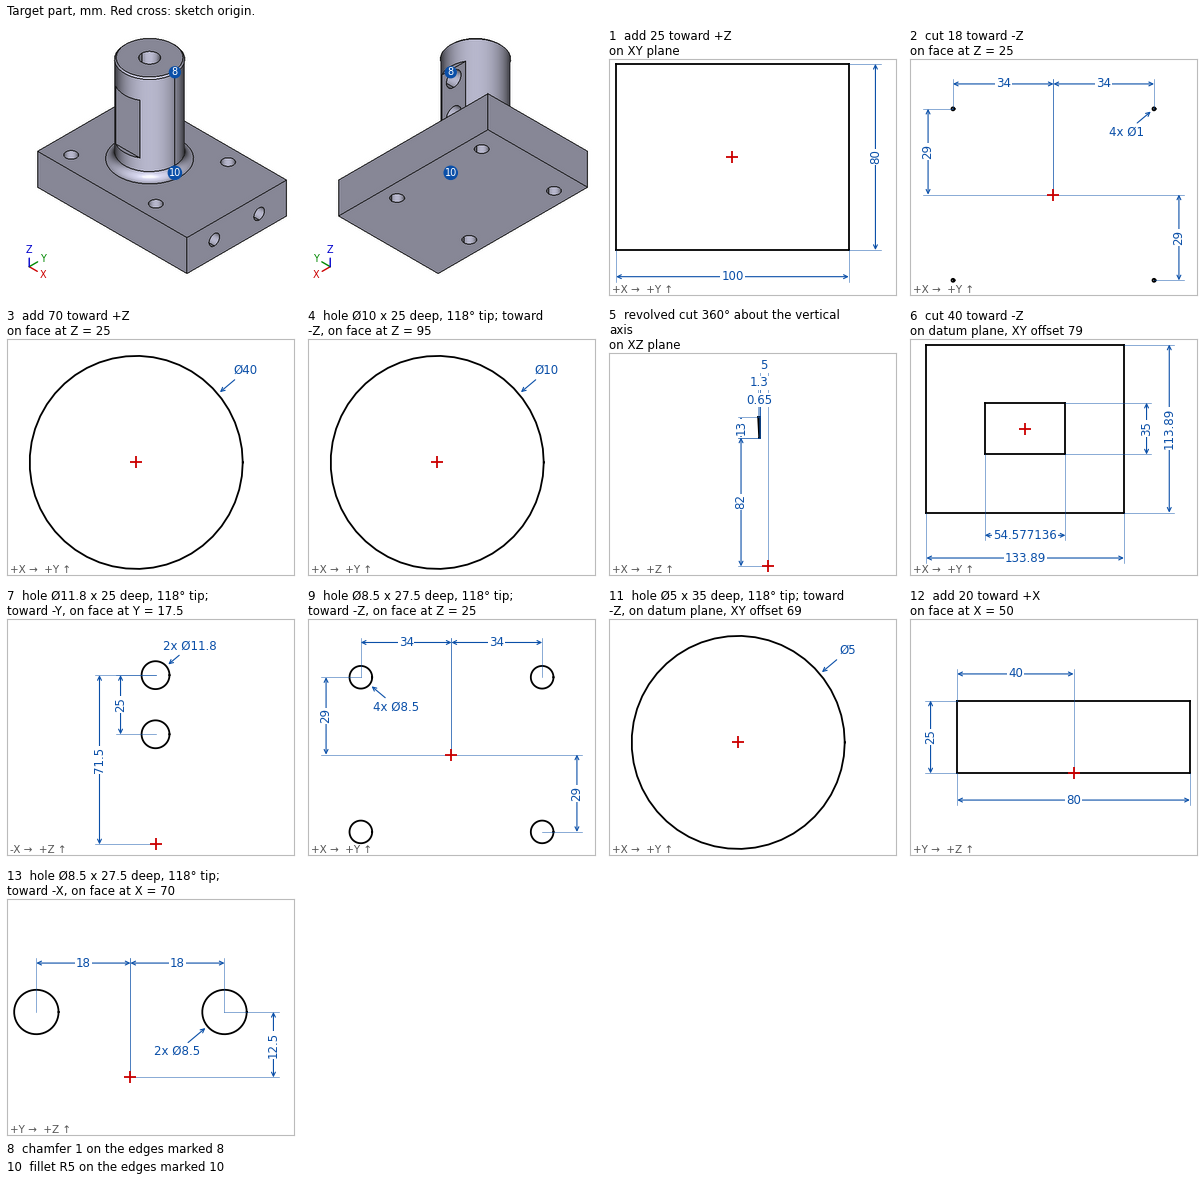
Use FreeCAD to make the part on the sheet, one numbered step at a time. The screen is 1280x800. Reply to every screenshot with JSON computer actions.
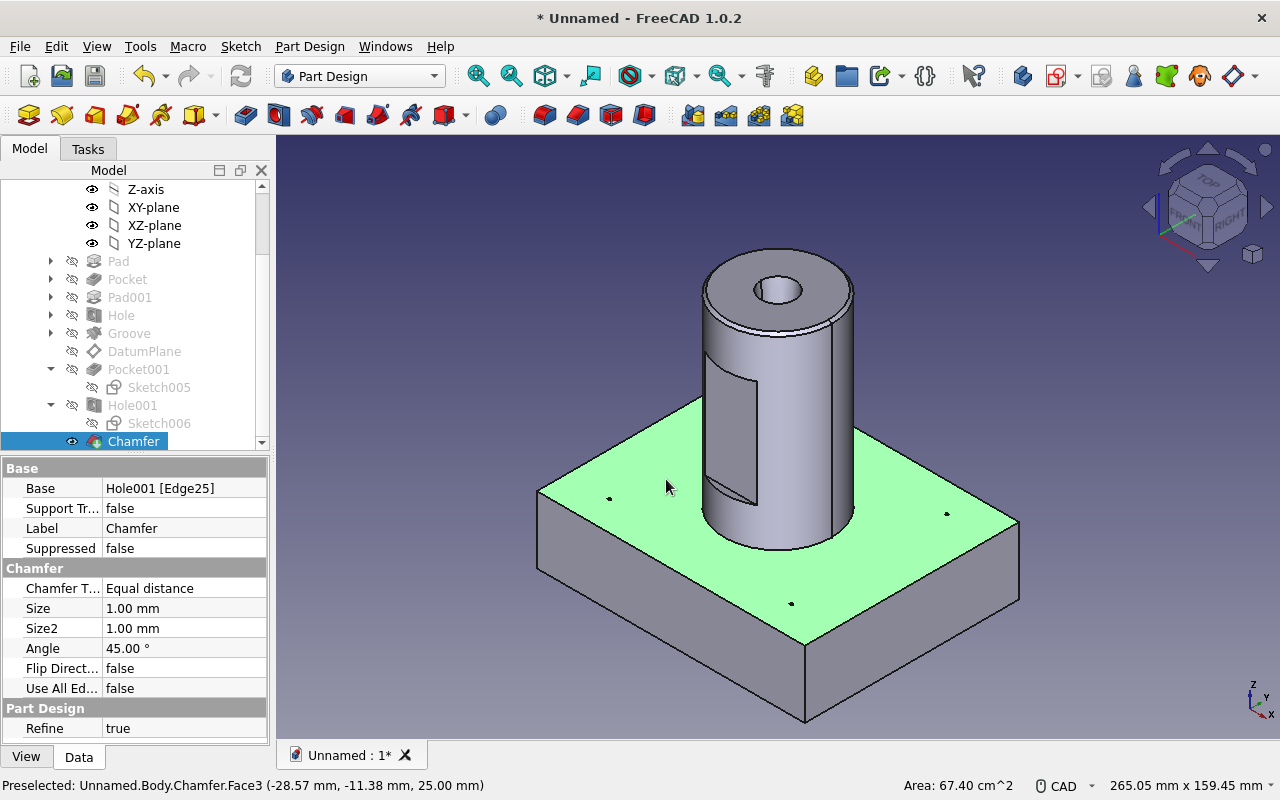
{"action": "left_click", "coordinate": [1056, 76]}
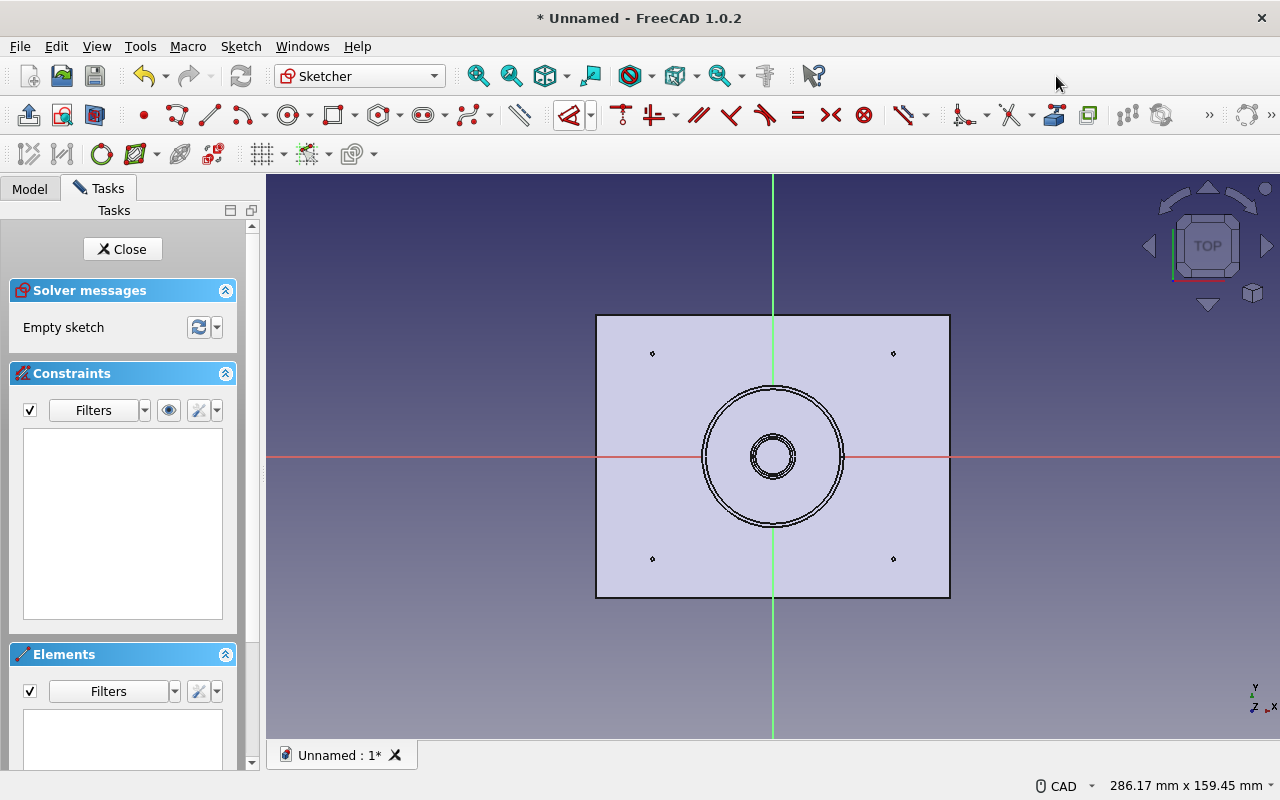
{"action": "scroll", "coordinate": [912, 456], "scroll_direction": "up", "scroll_amount": 2}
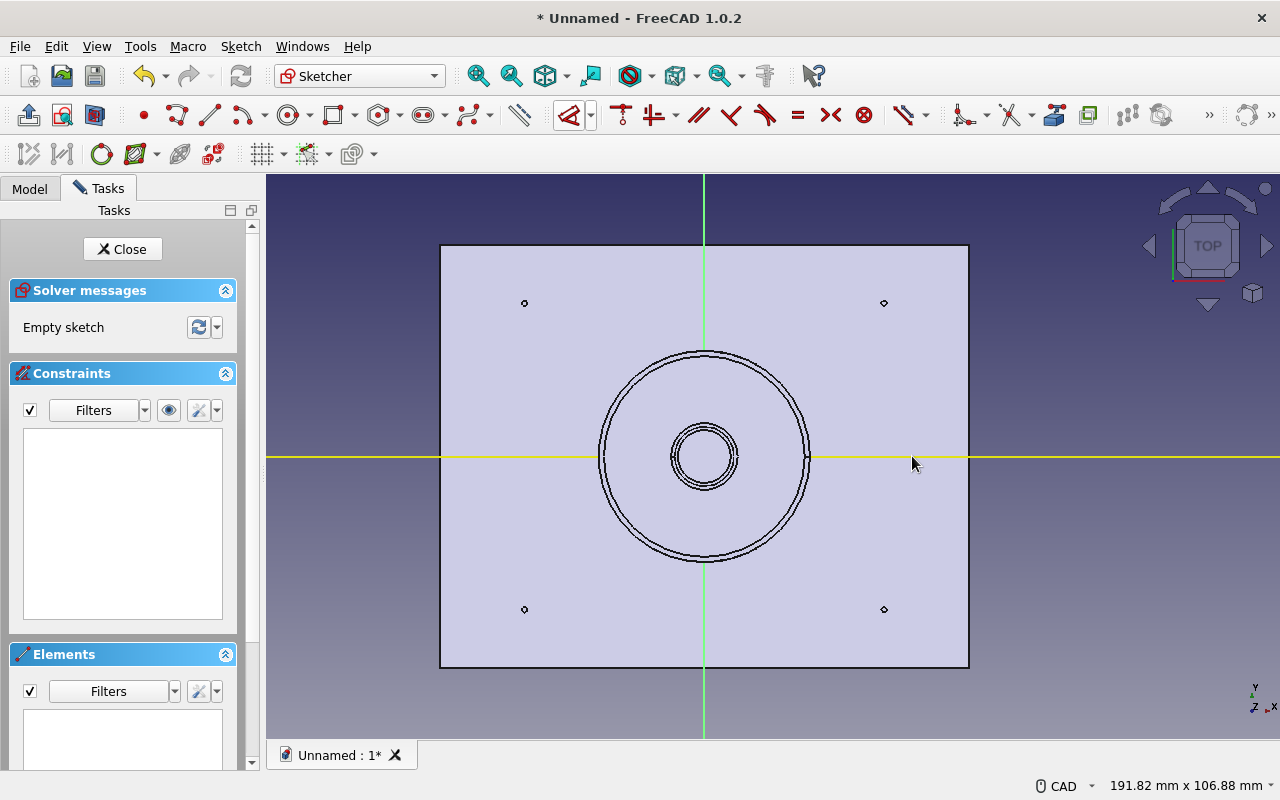
{"action": "key", "text": "g c"}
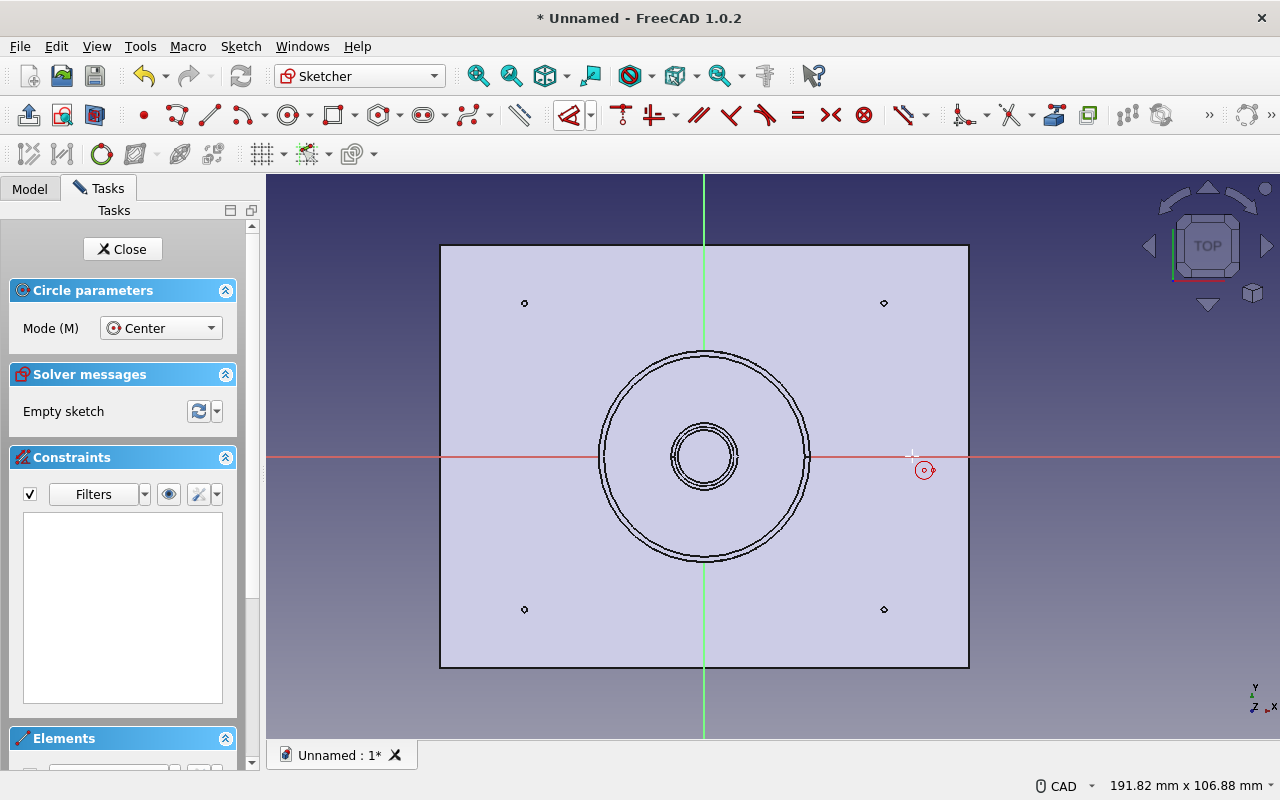
{"action": "left_click", "coordinate": [525, 303]}
{"action": "mouse_move", "coordinate": [540, 287]}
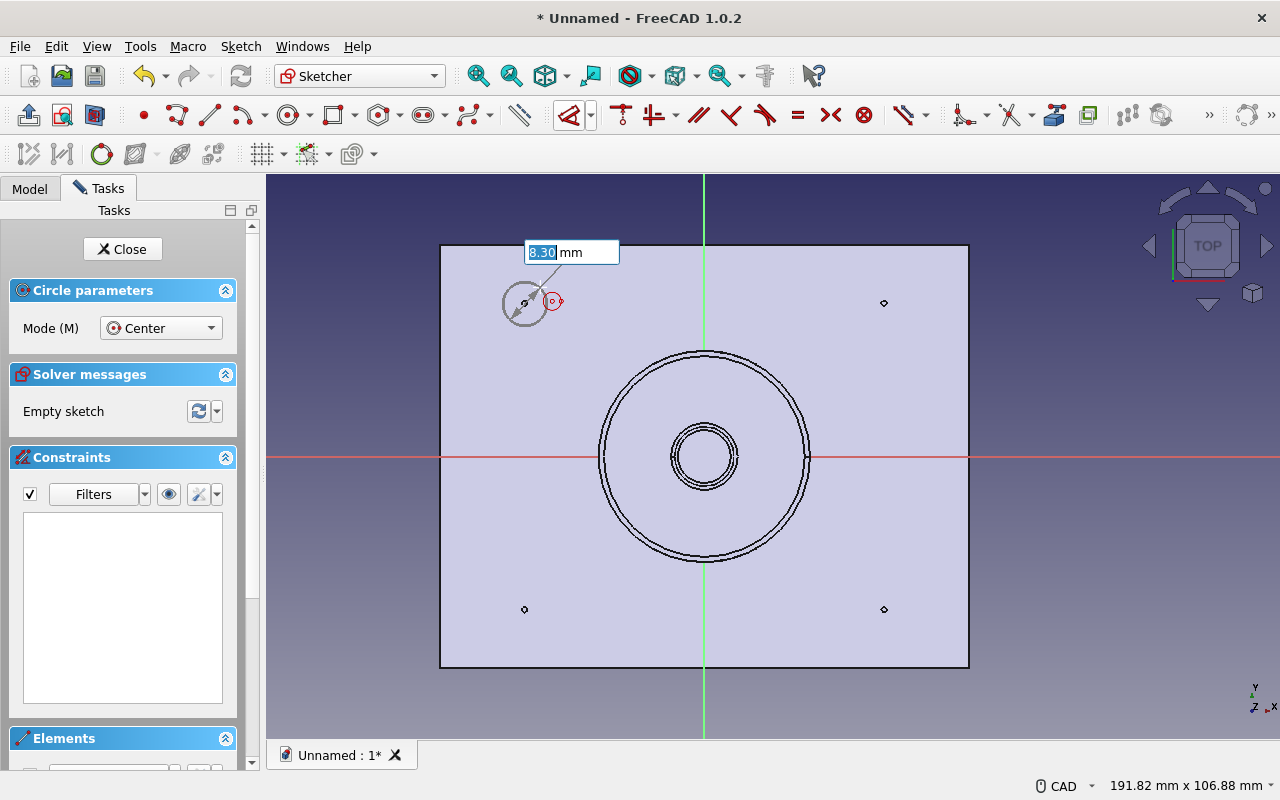
{"action": "type", "text": "8.5"}
{"action": "key", "text": "Return"}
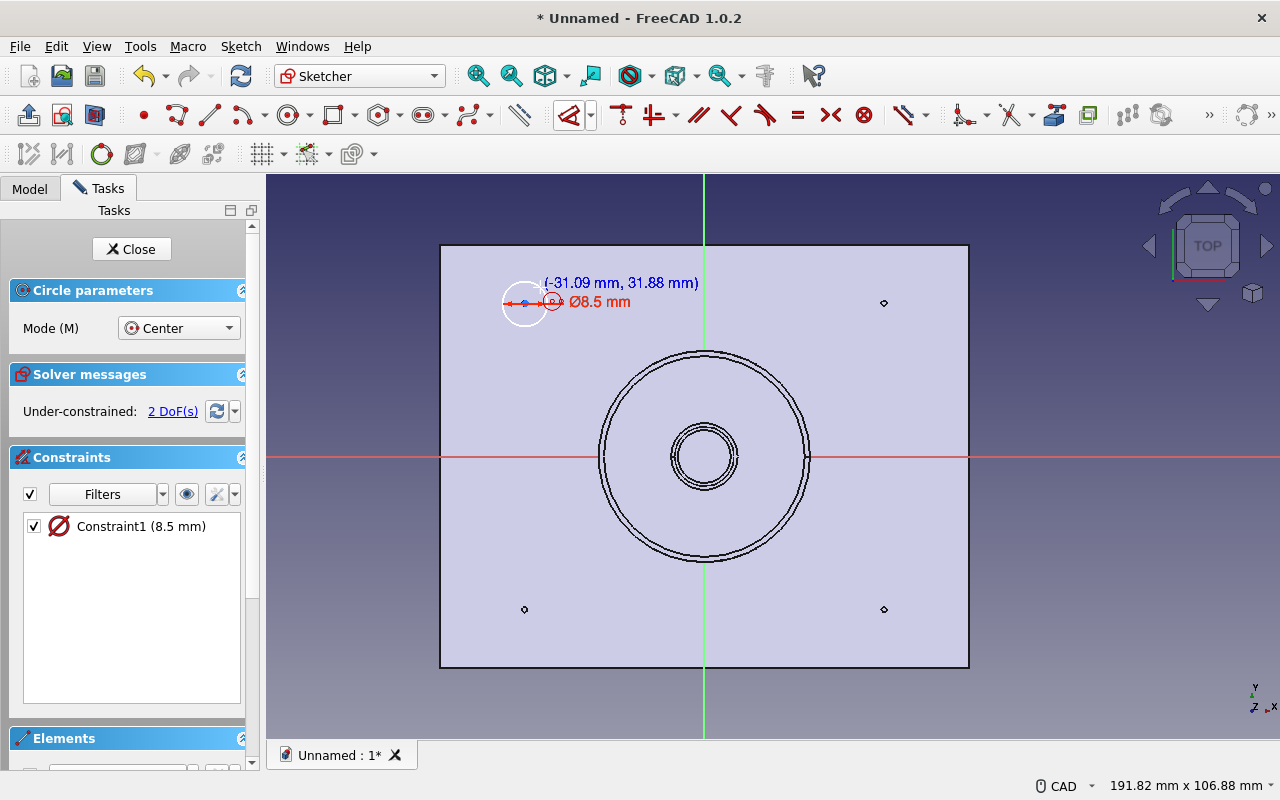
{"action": "left_click", "coordinate": [884, 303]}
{"action": "mouse_move", "coordinate": [900, 287]}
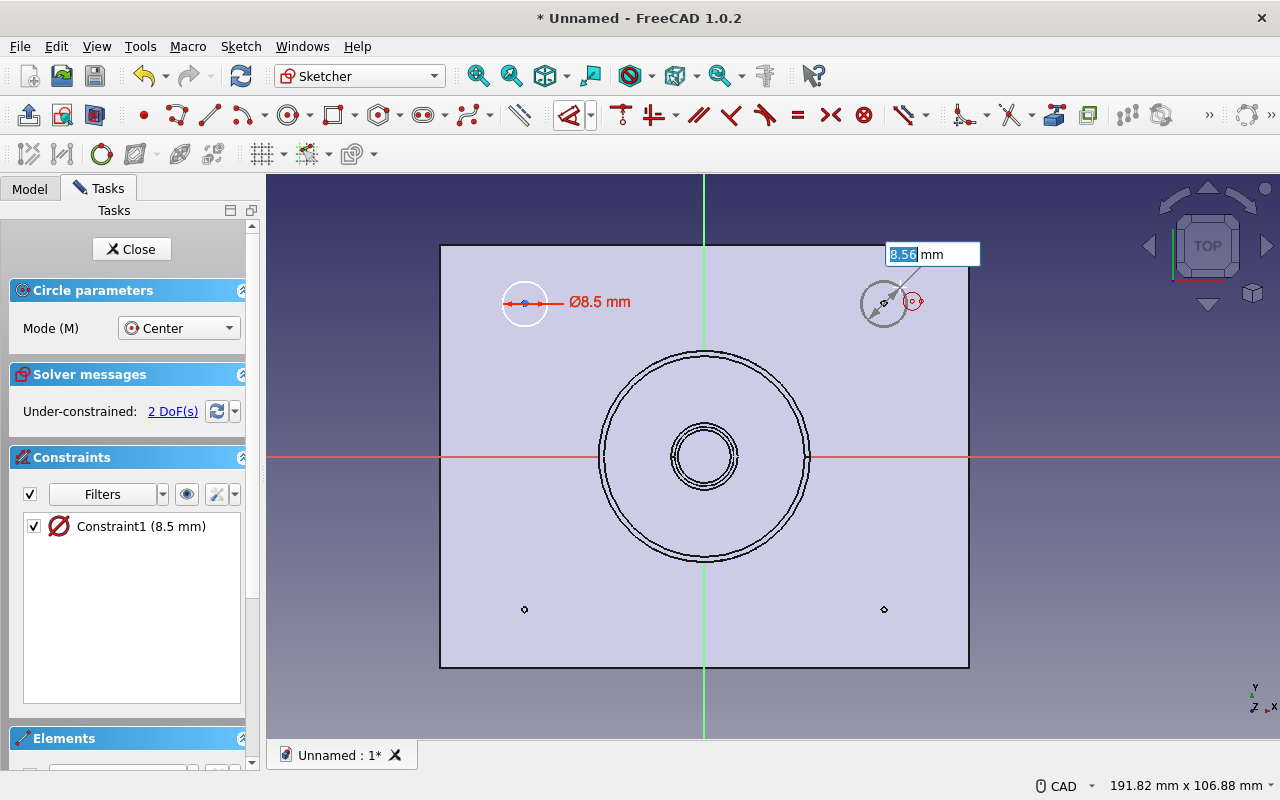
{"action": "type", "text": "8.5"}
{"action": "key", "text": "Return"}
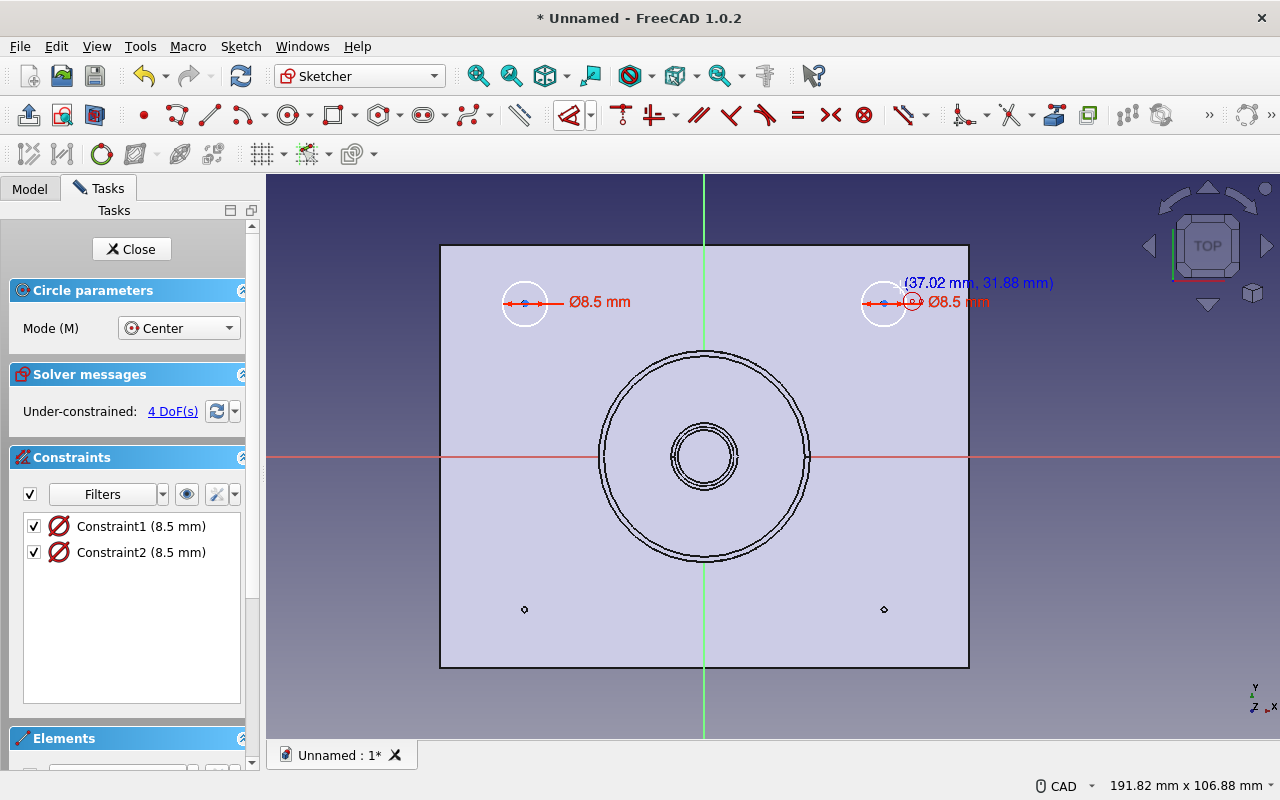
{"action": "left_click", "coordinate": [884, 610]}
{"action": "mouse_move", "coordinate": [900, 594]}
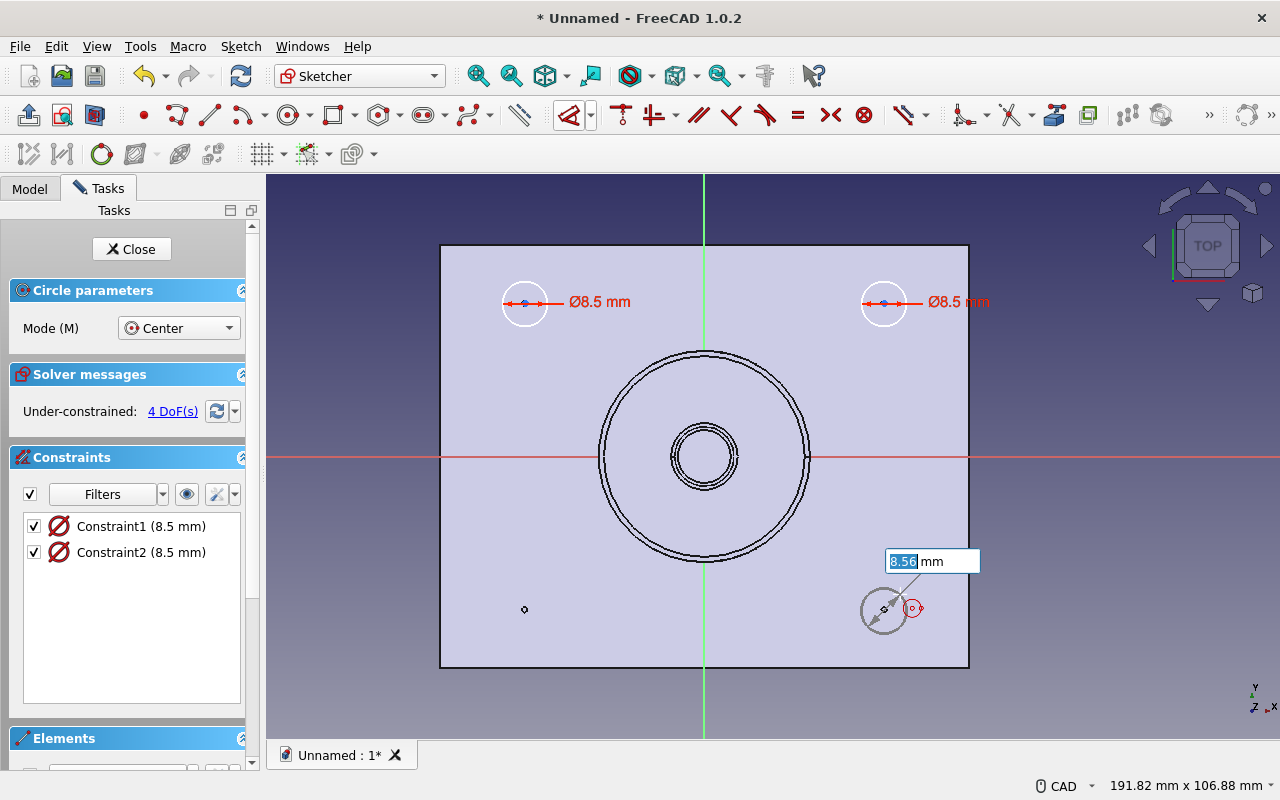
{"action": "type", "text": "8.5"}
{"action": "key", "text": "Return"}